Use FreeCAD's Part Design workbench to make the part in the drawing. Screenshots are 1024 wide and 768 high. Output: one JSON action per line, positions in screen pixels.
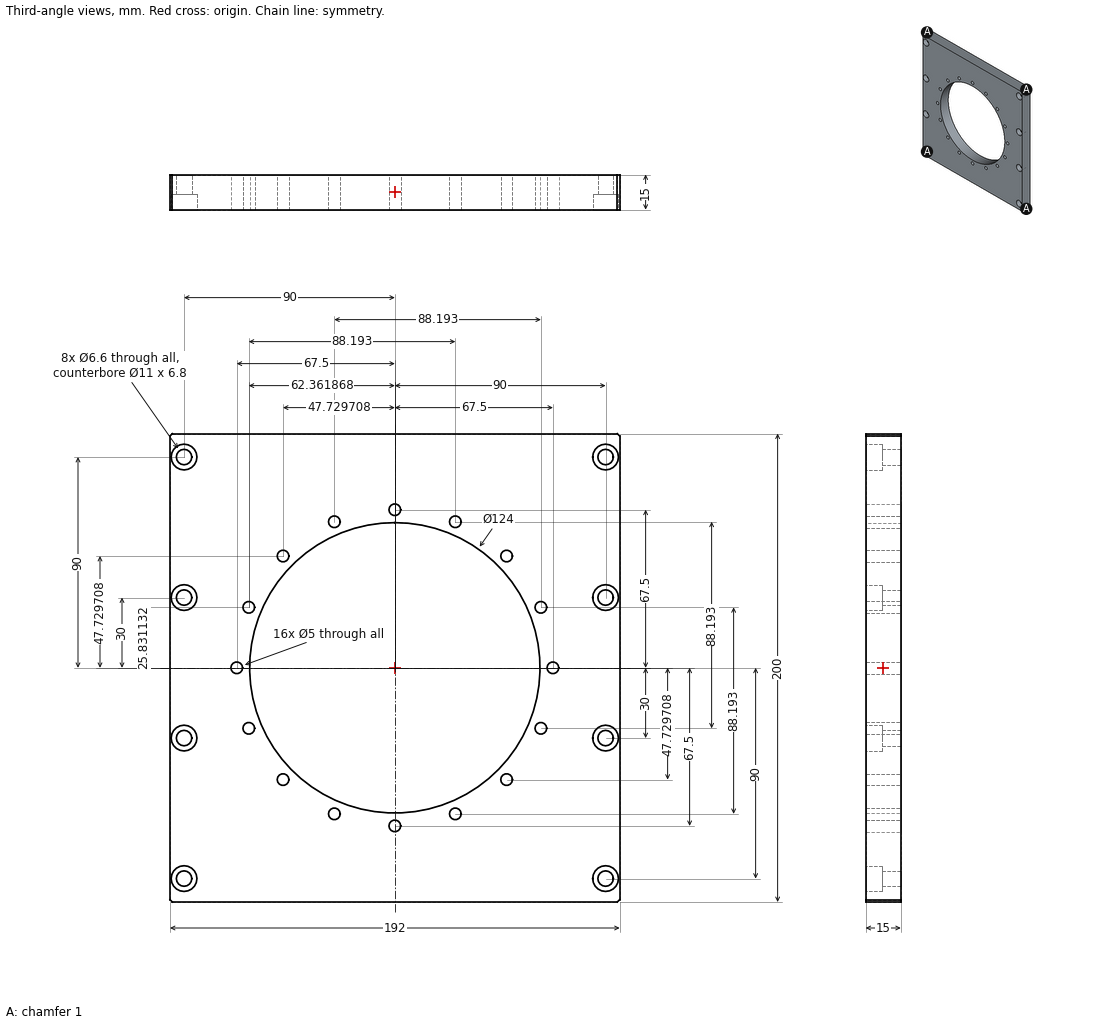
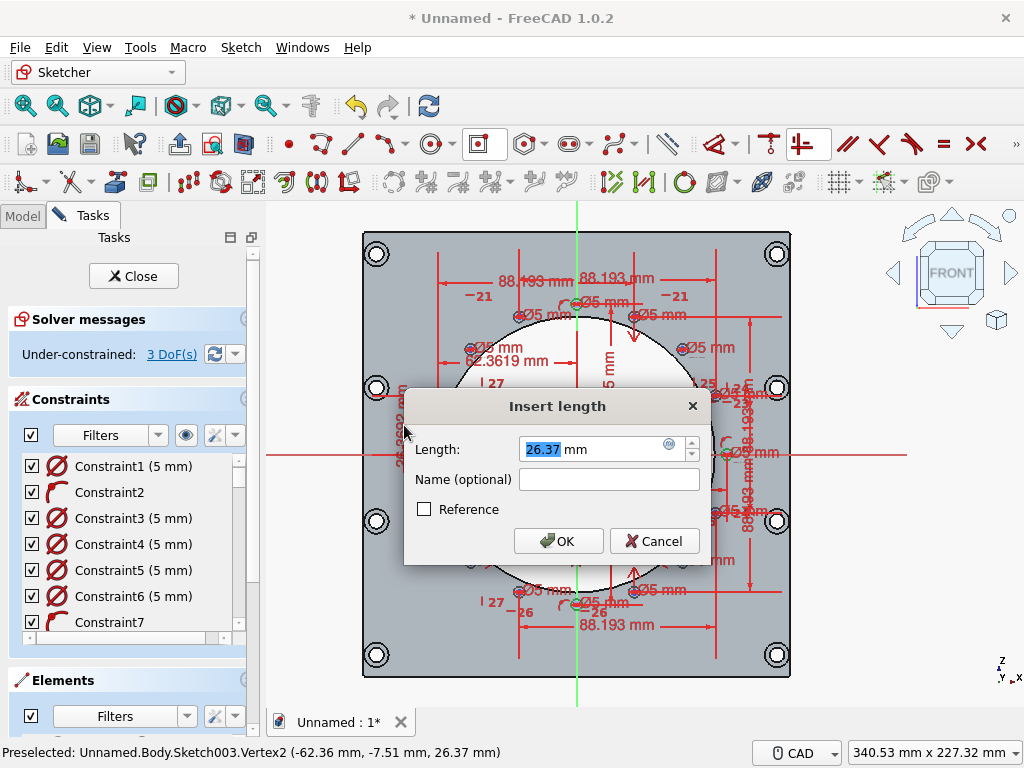
{"action": "type", "text": "25.831132"}
{"action": "key", "text": "Return"}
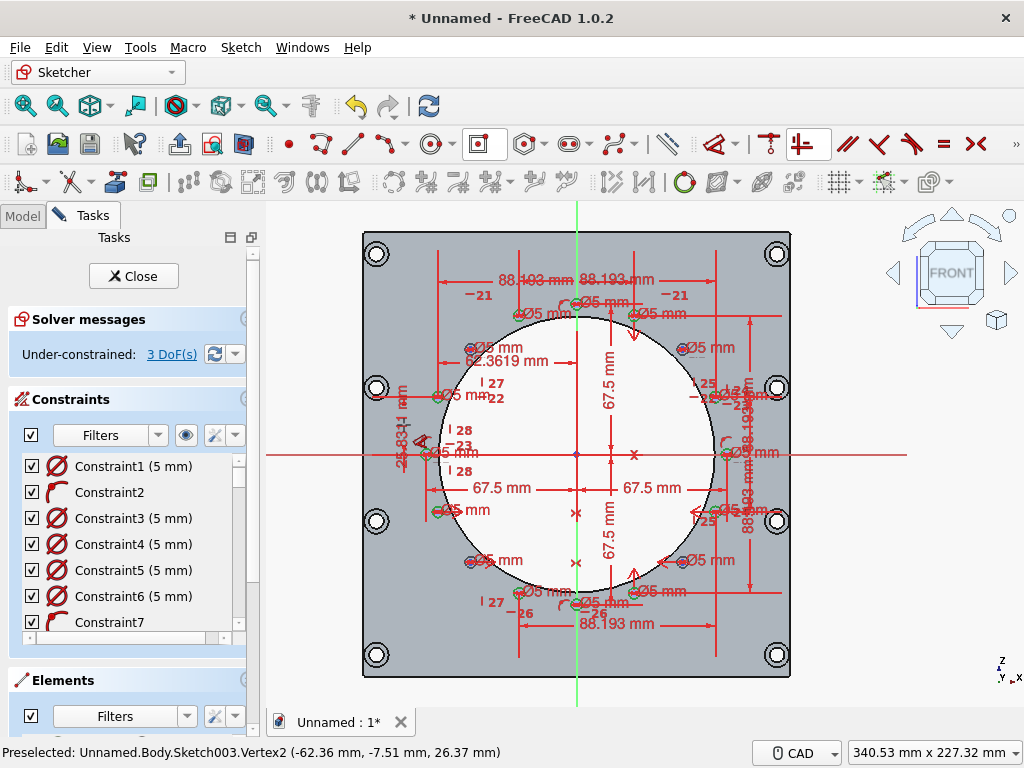
{"action": "left_click", "coordinate": [471, 350]}
{"action": "left_click", "coordinate": [499, 316]}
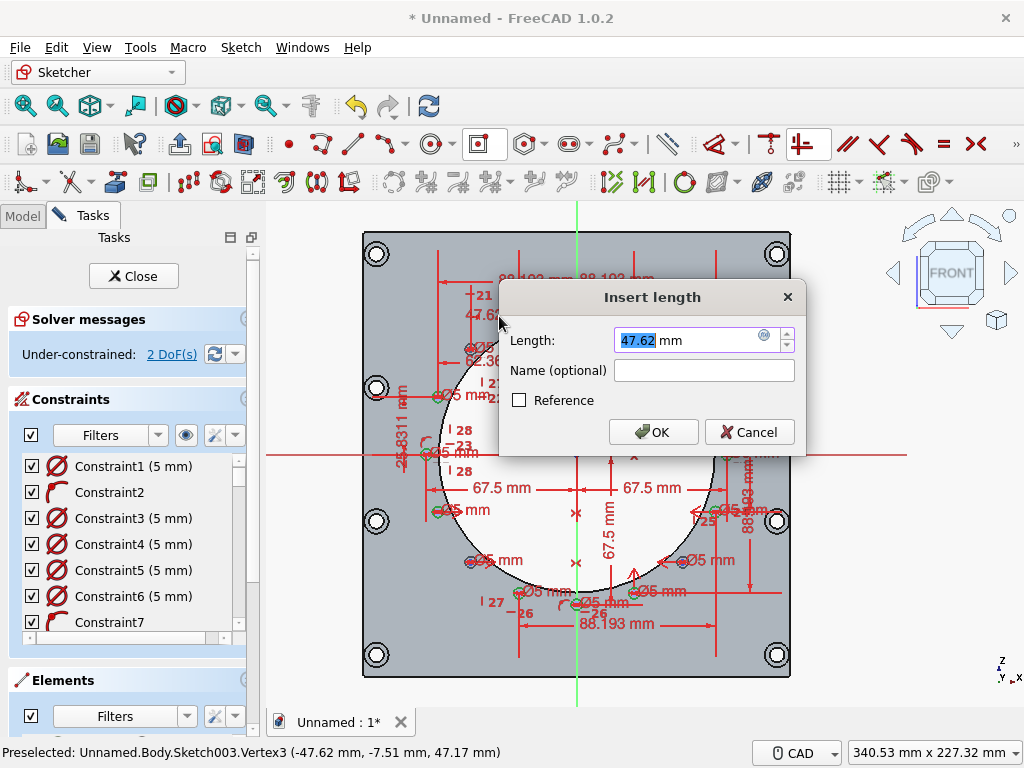
{"action": "type", "text": "47.729708"}
{"action": "key", "text": "Return"}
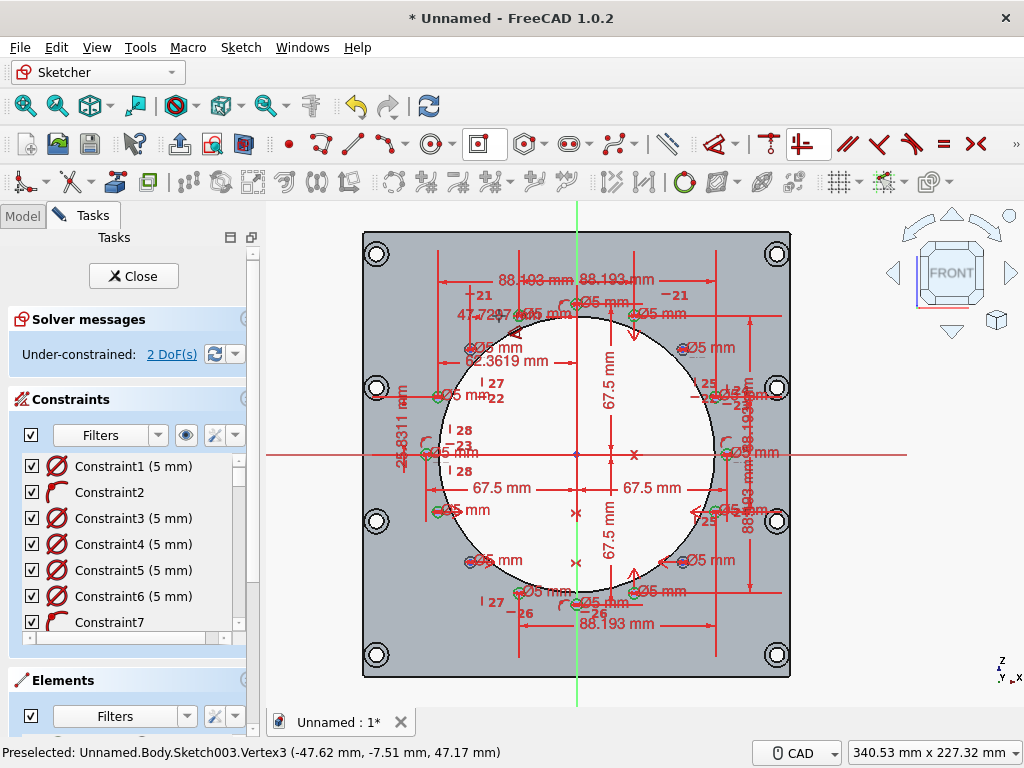
{"action": "left_click", "coordinate": [471, 350]}
{"action": "left_click", "coordinate": [437, 378]}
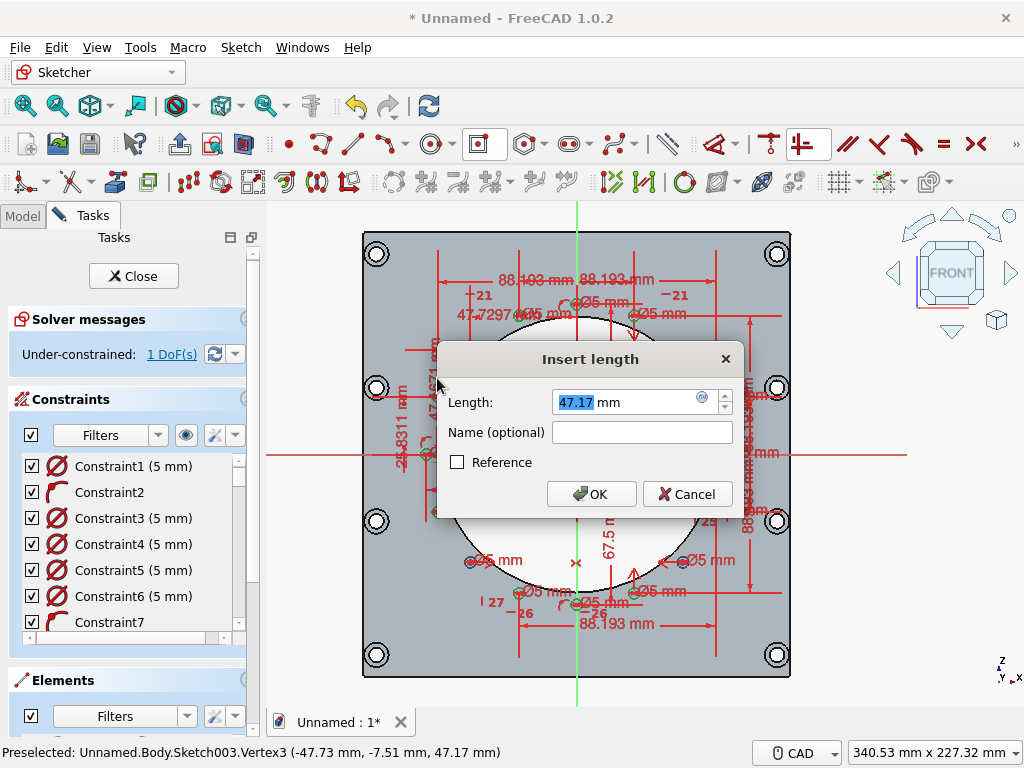
{"action": "type", "text": "47.729708"}
{"action": "key", "text": "Return"}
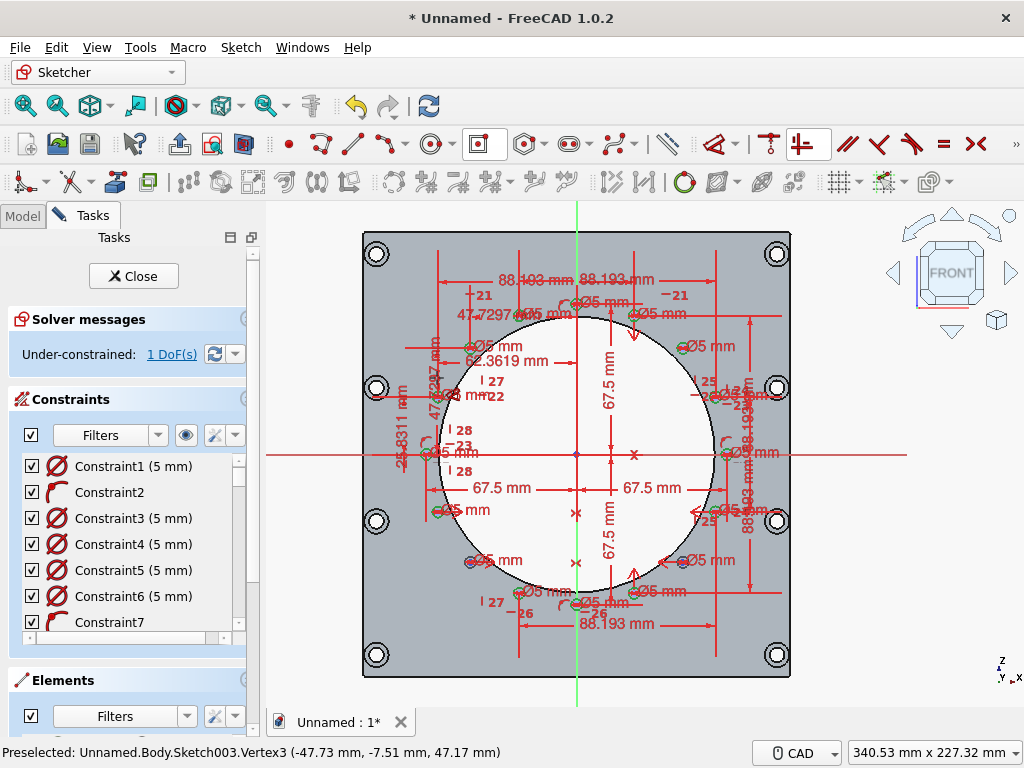
{"action": "left_click", "coordinate": [683, 562]}
{"action": "left_click", "coordinate": [717, 533]}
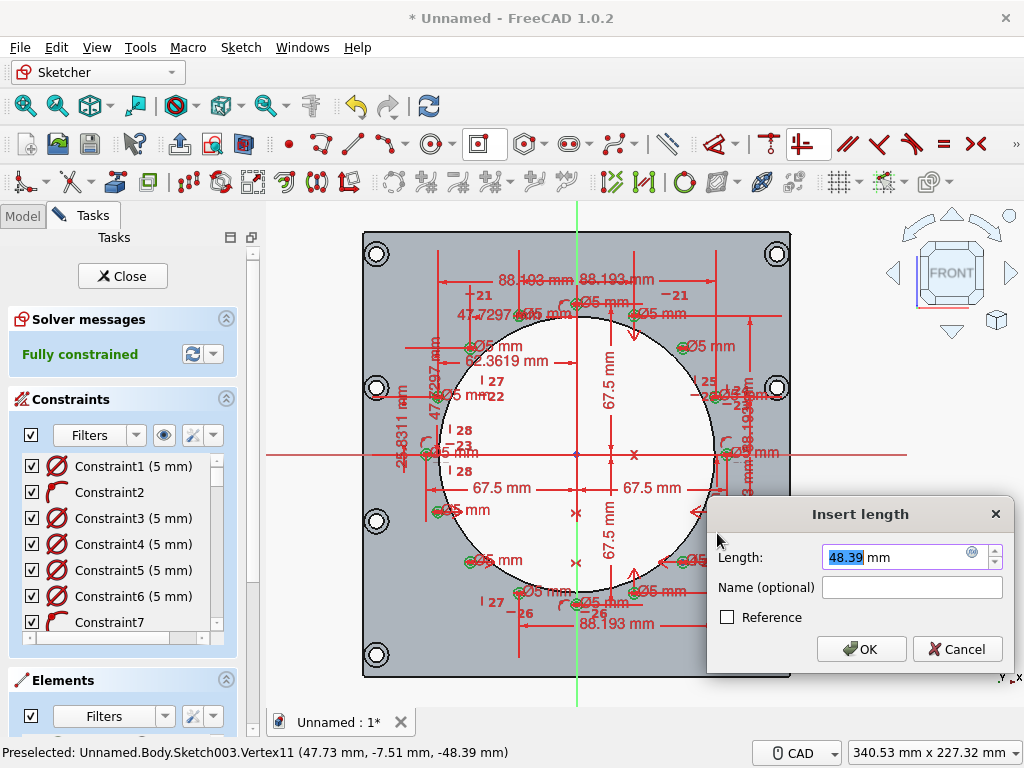
{"action": "type", "text": "47.729708"}
{"action": "key", "text": "Return"}
{"action": "key", "text": "Escape"}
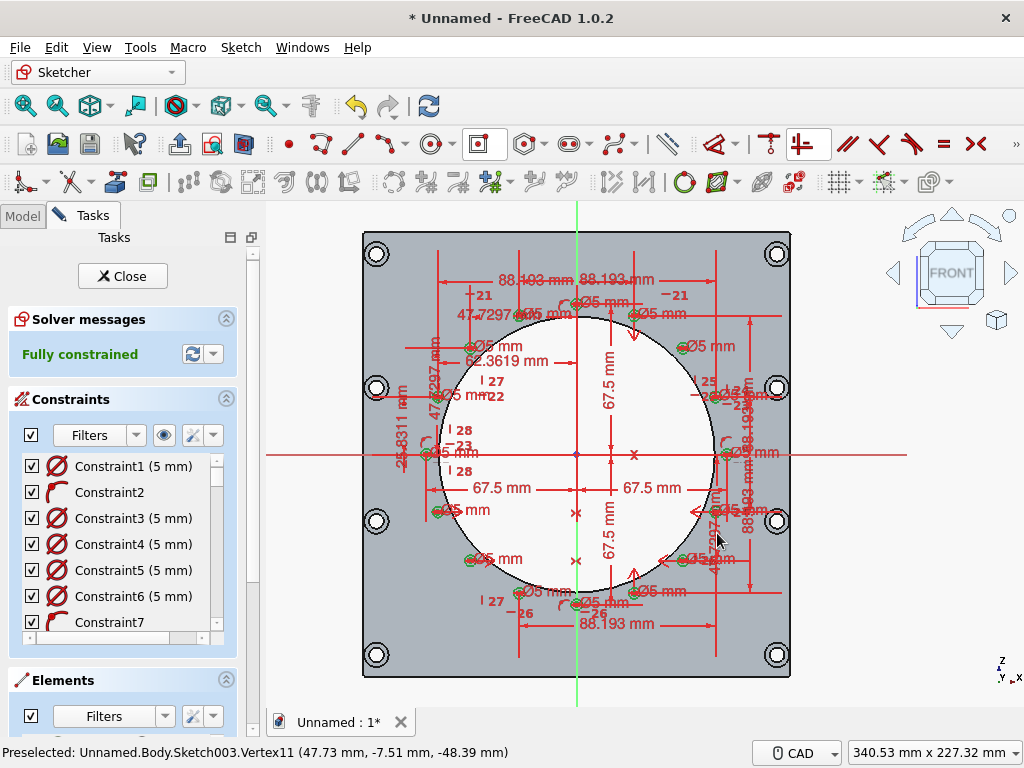
{"action": "left_click", "coordinate": [123, 276]}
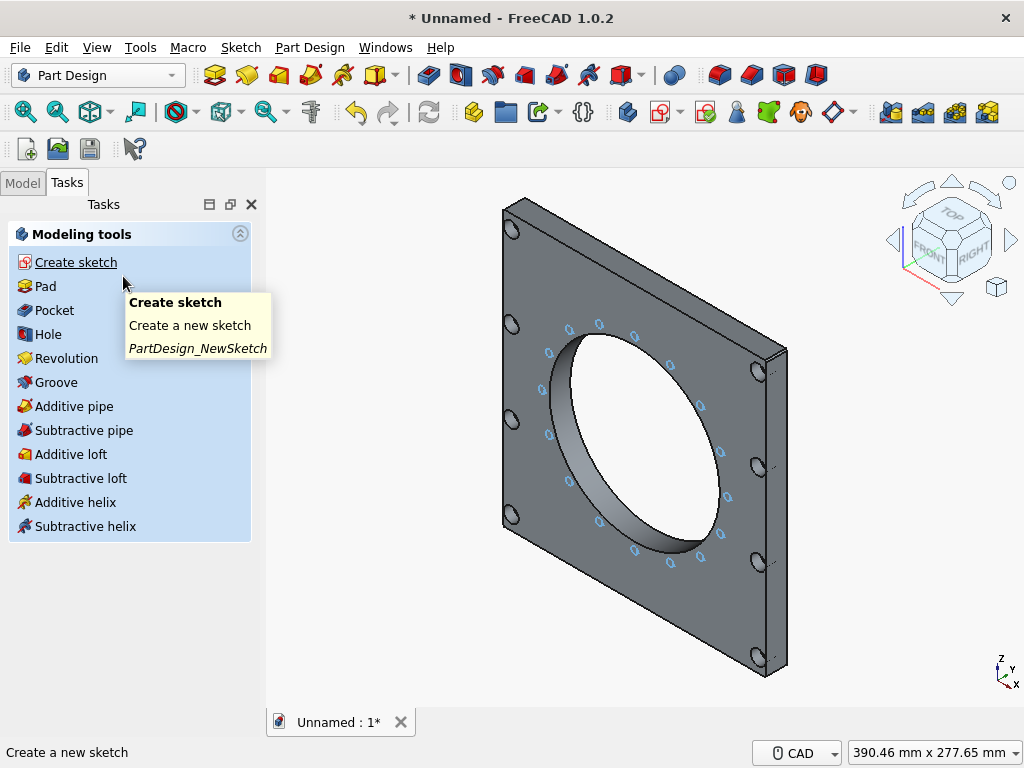
{"action": "left_click", "coordinate": [462, 76]}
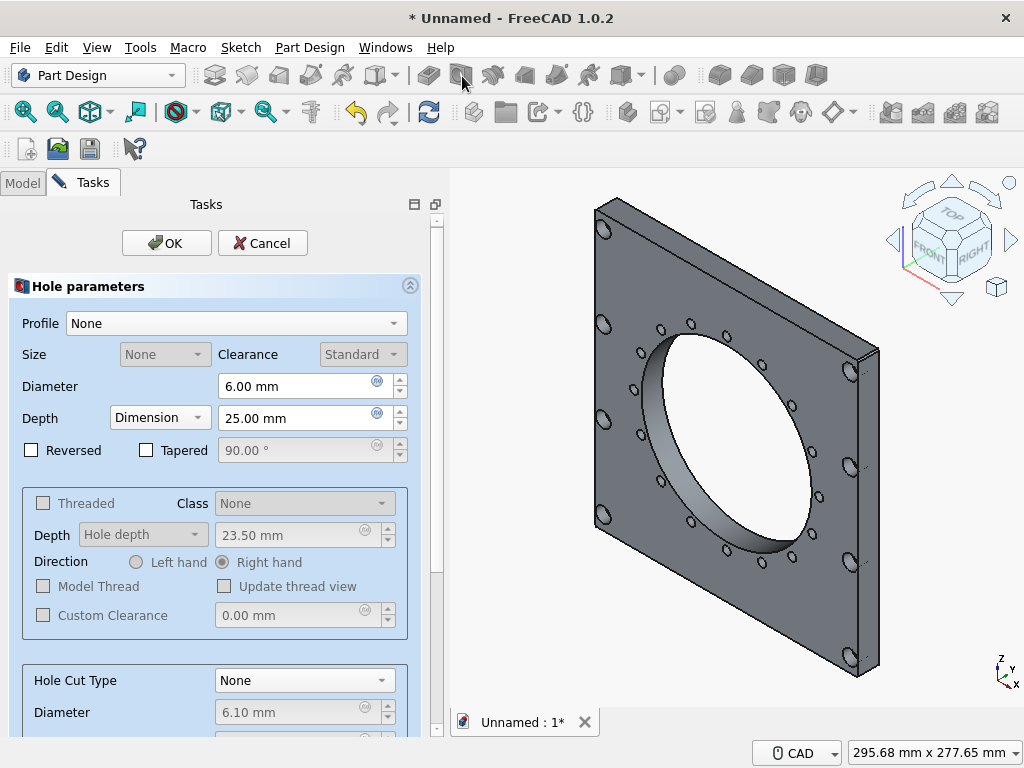
{"action": "triple_click", "coordinate": [305, 386]}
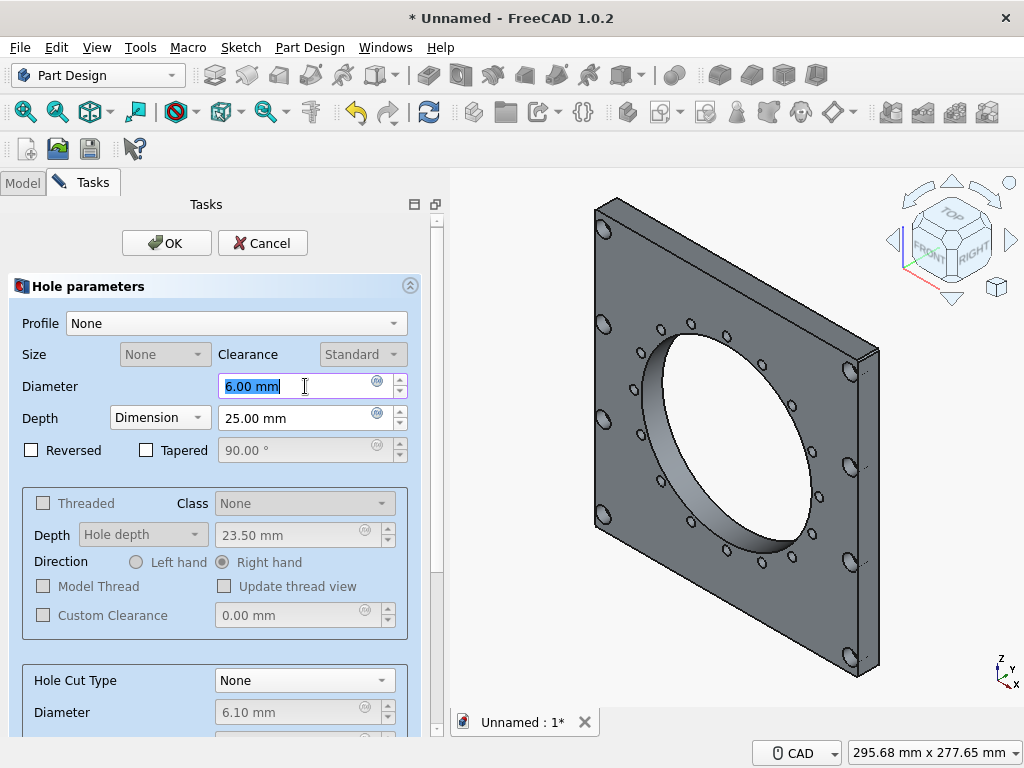
{"action": "type", "text": "5"}
{"action": "key", "text": "Tab"}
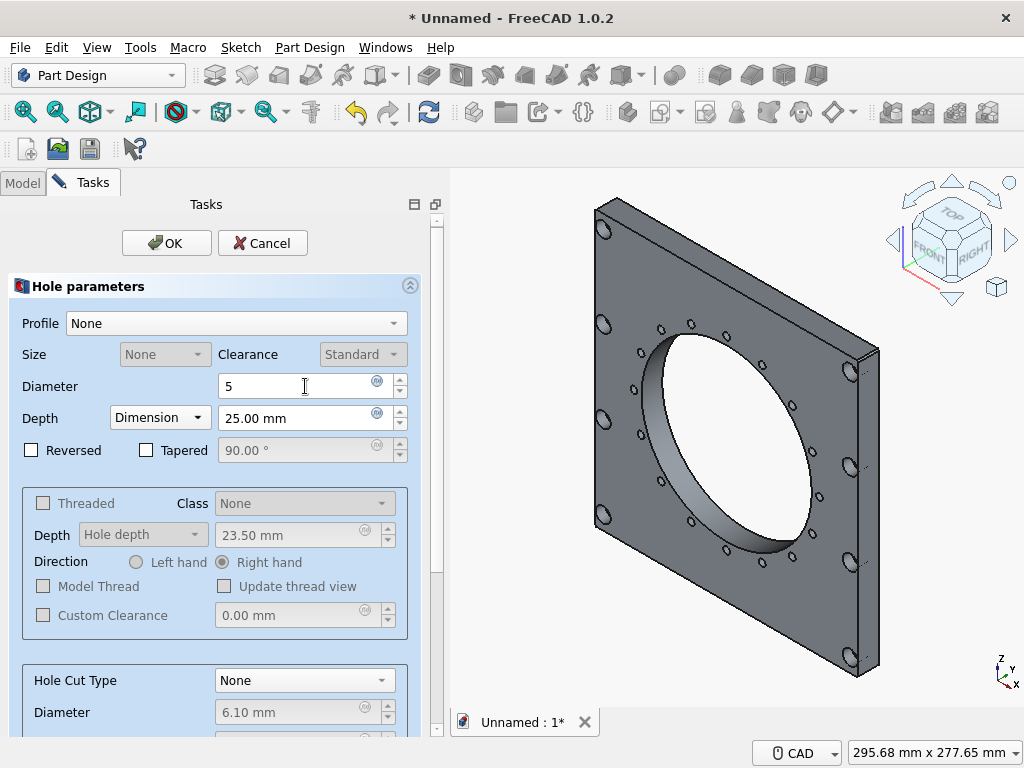
{"action": "left_click", "coordinate": [161, 418]}